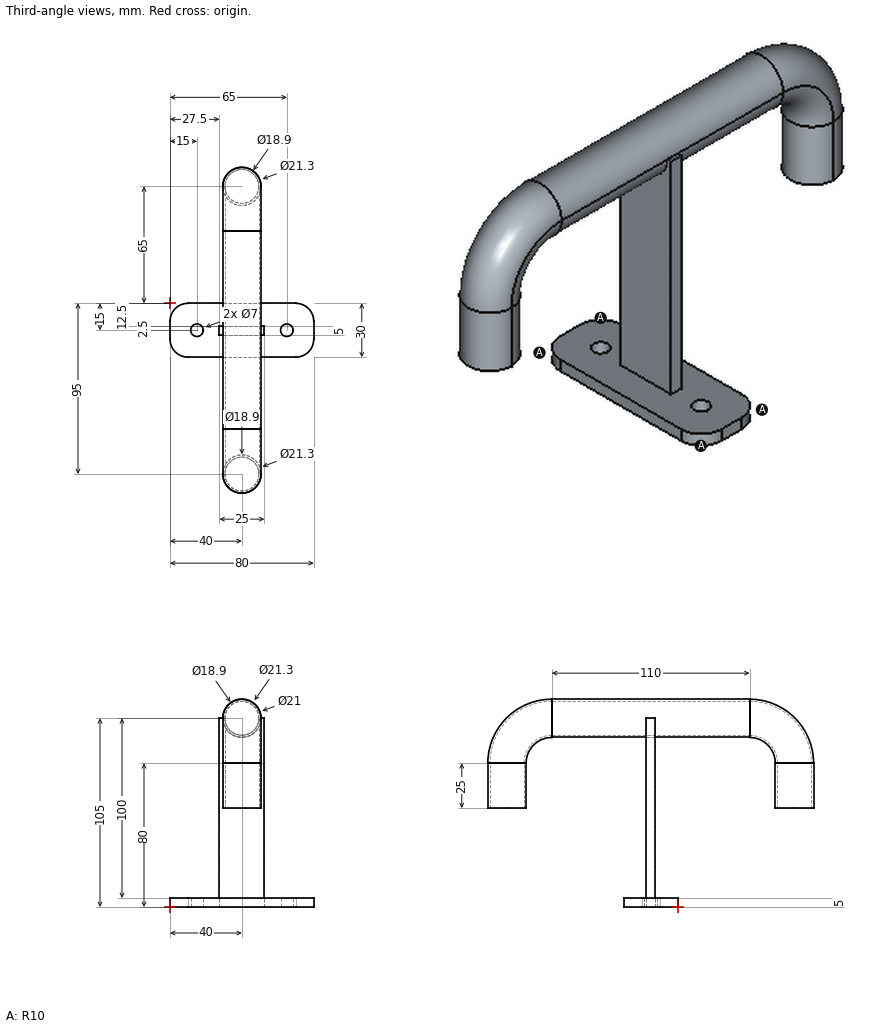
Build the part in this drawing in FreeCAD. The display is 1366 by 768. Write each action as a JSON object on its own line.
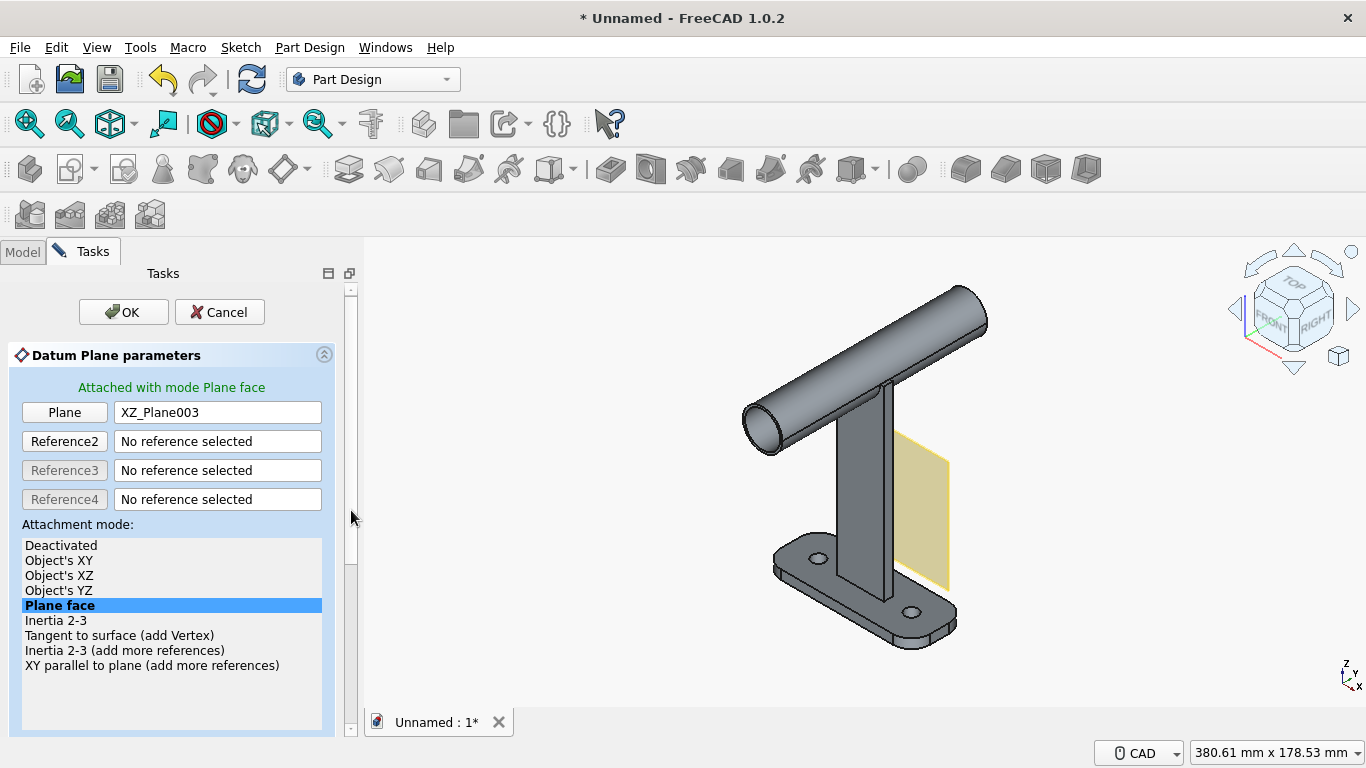
{"action": "left_click", "coordinate": [124, 312]}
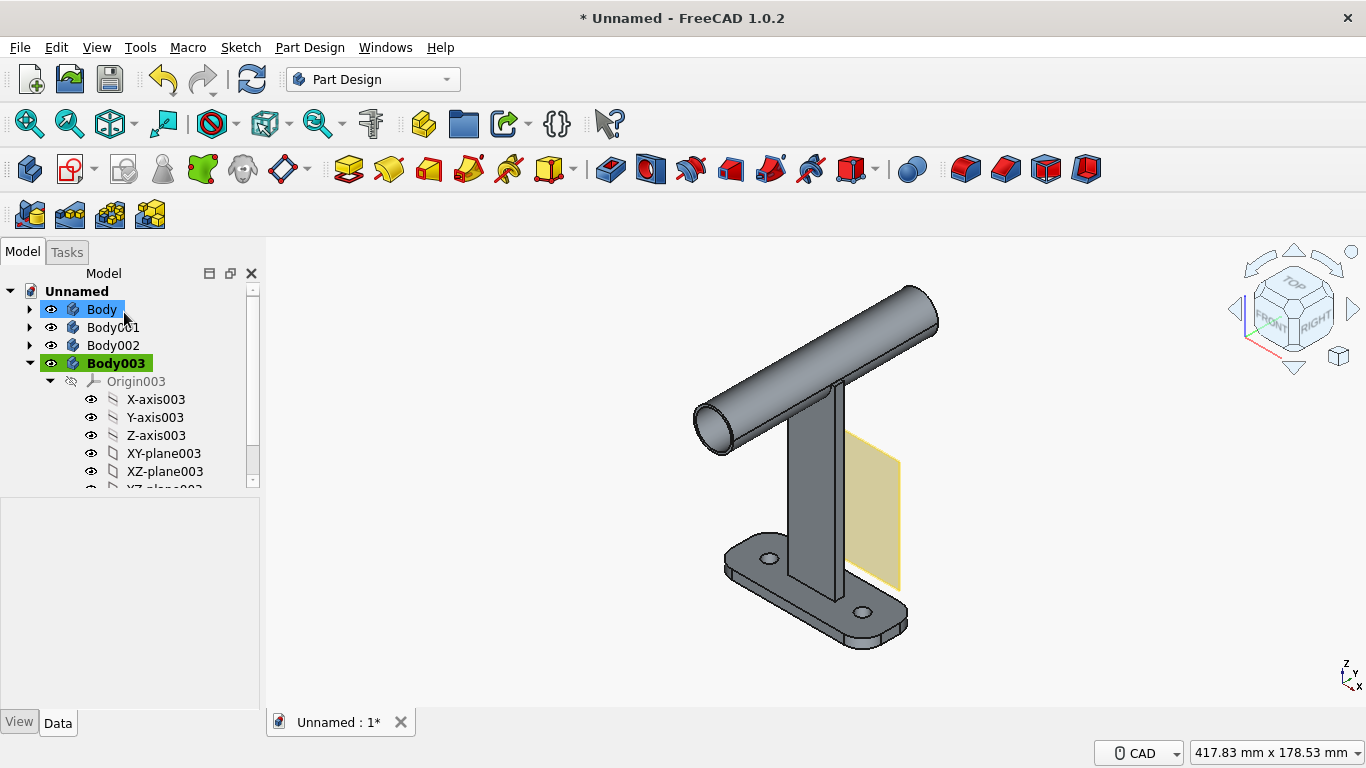
{"action": "scroll", "coordinate": [100, 377], "scroll_direction": "down", "scroll_amount": 3}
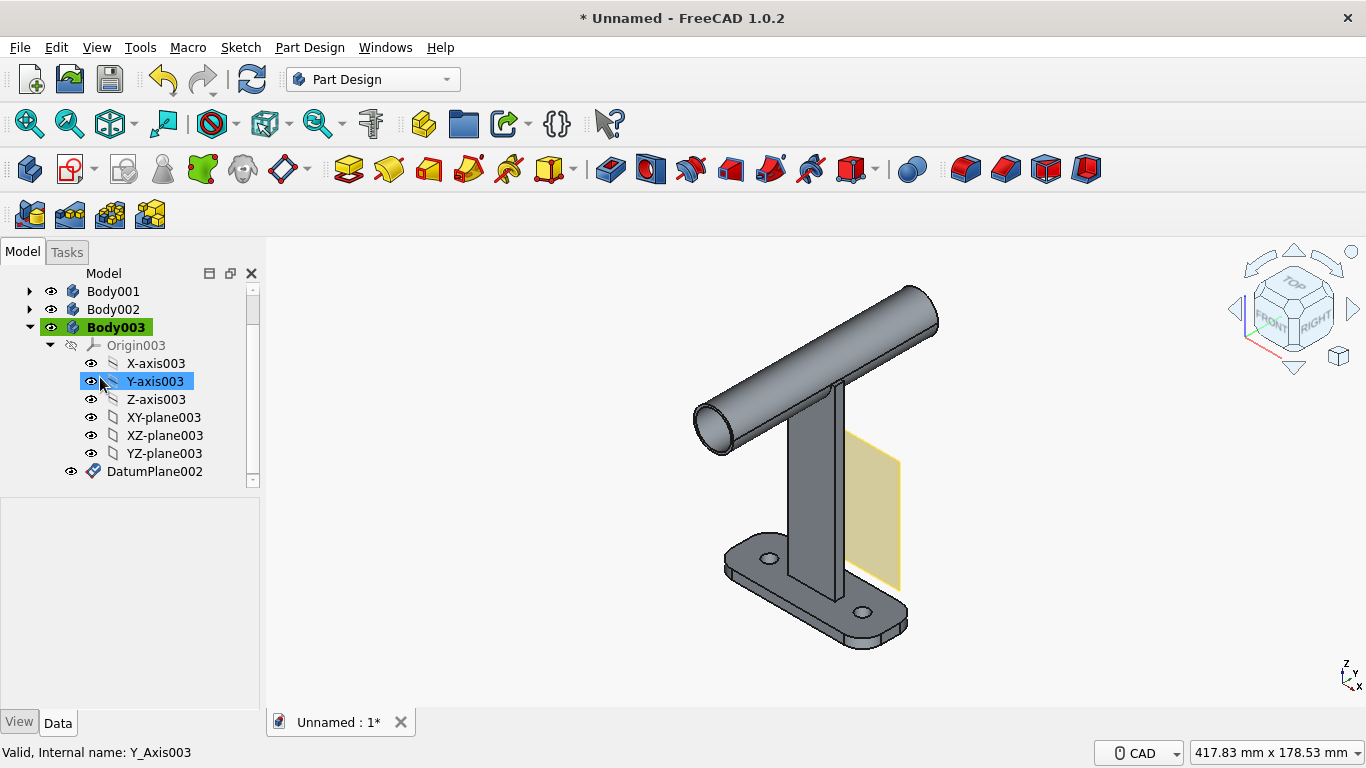
{"action": "left_click", "coordinate": [116, 471]}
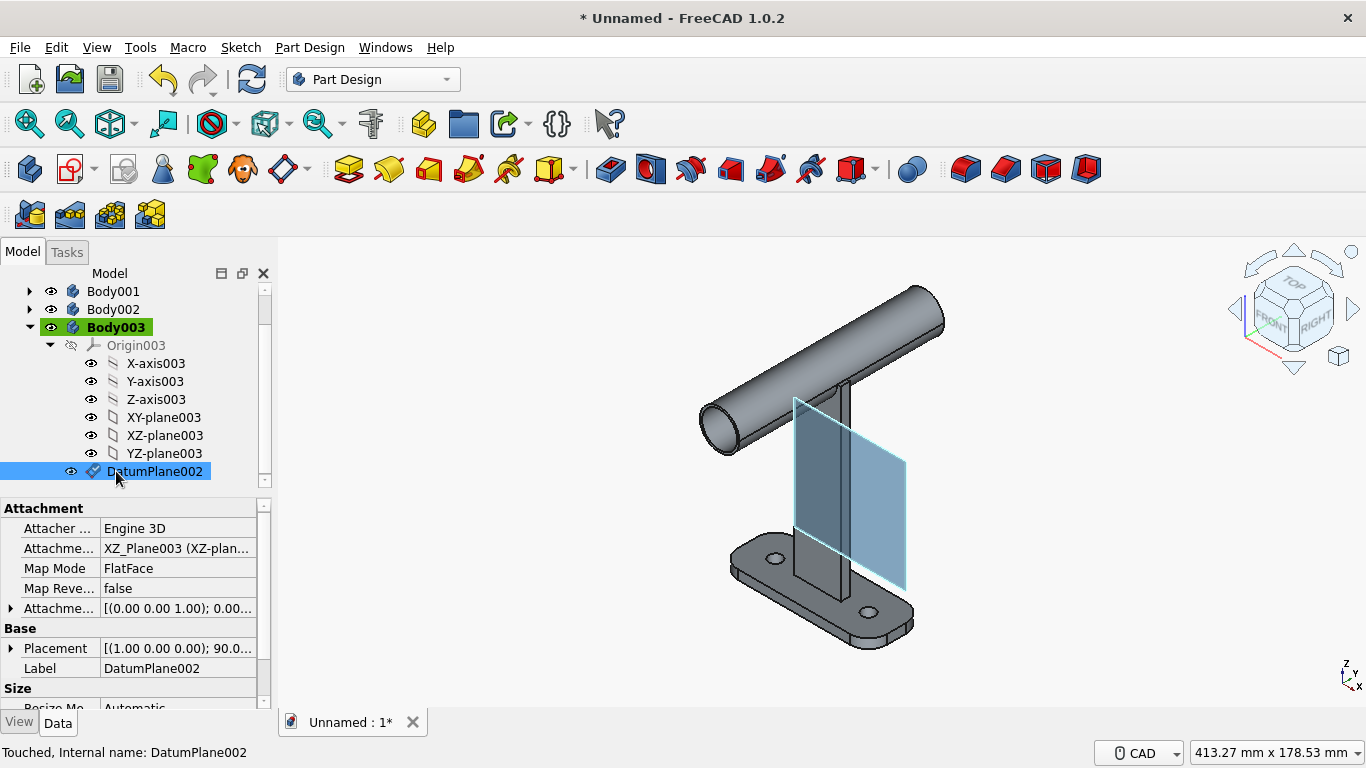
{"action": "left_click", "coordinate": [70, 170]}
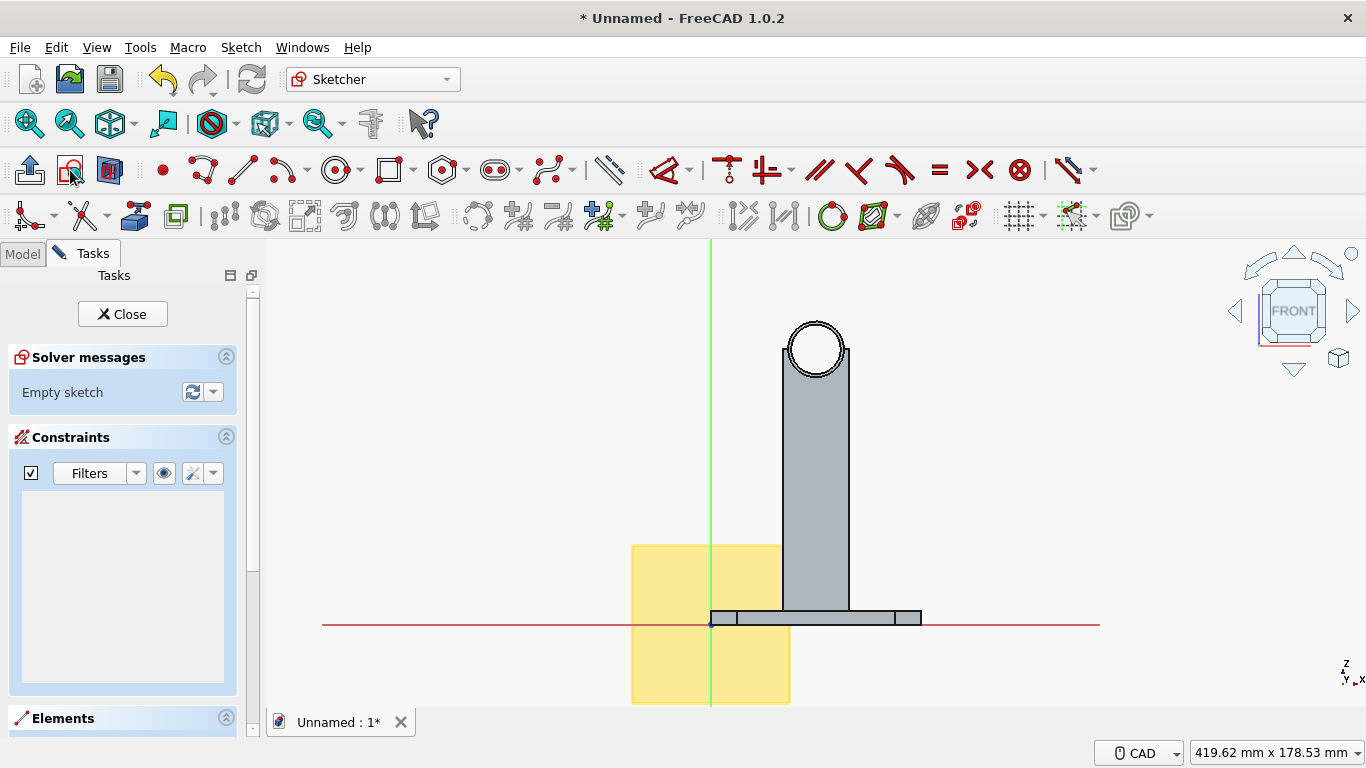
{"action": "scroll", "coordinate": [846, 323], "scroll_direction": "up", "scroll_amount": 6}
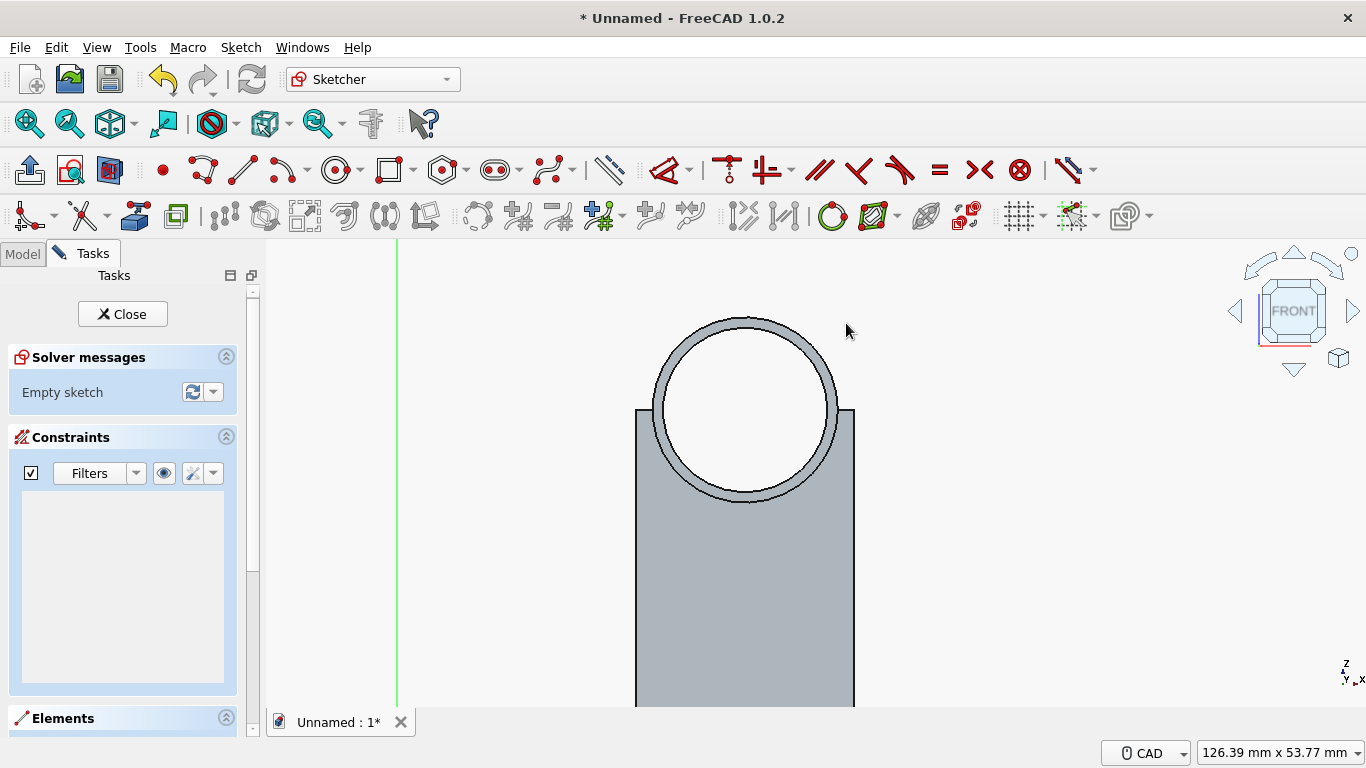
{"action": "left_click", "coordinate": [336, 170]}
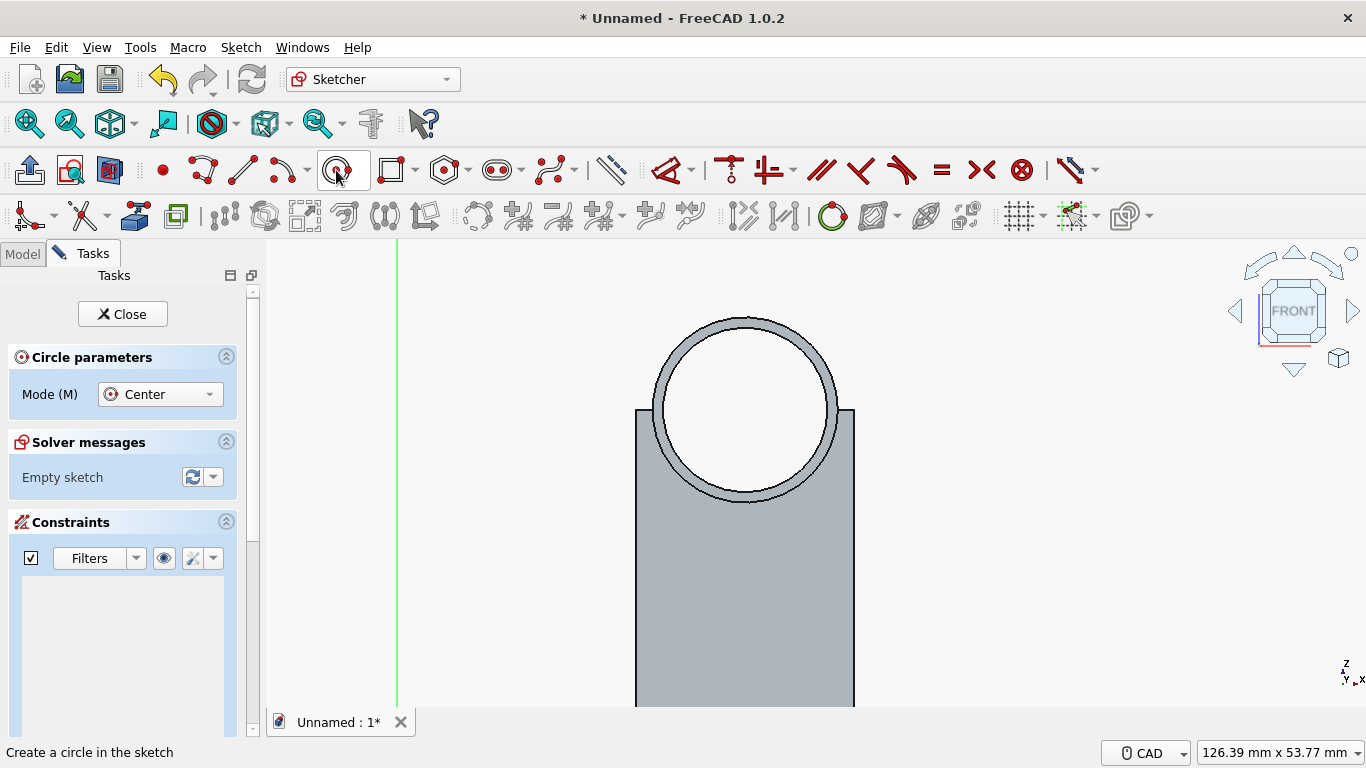
{"action": "left_click", "coordinate": [745, 410]}
{"action": "mouse_move", "coordinate": [811, 344]}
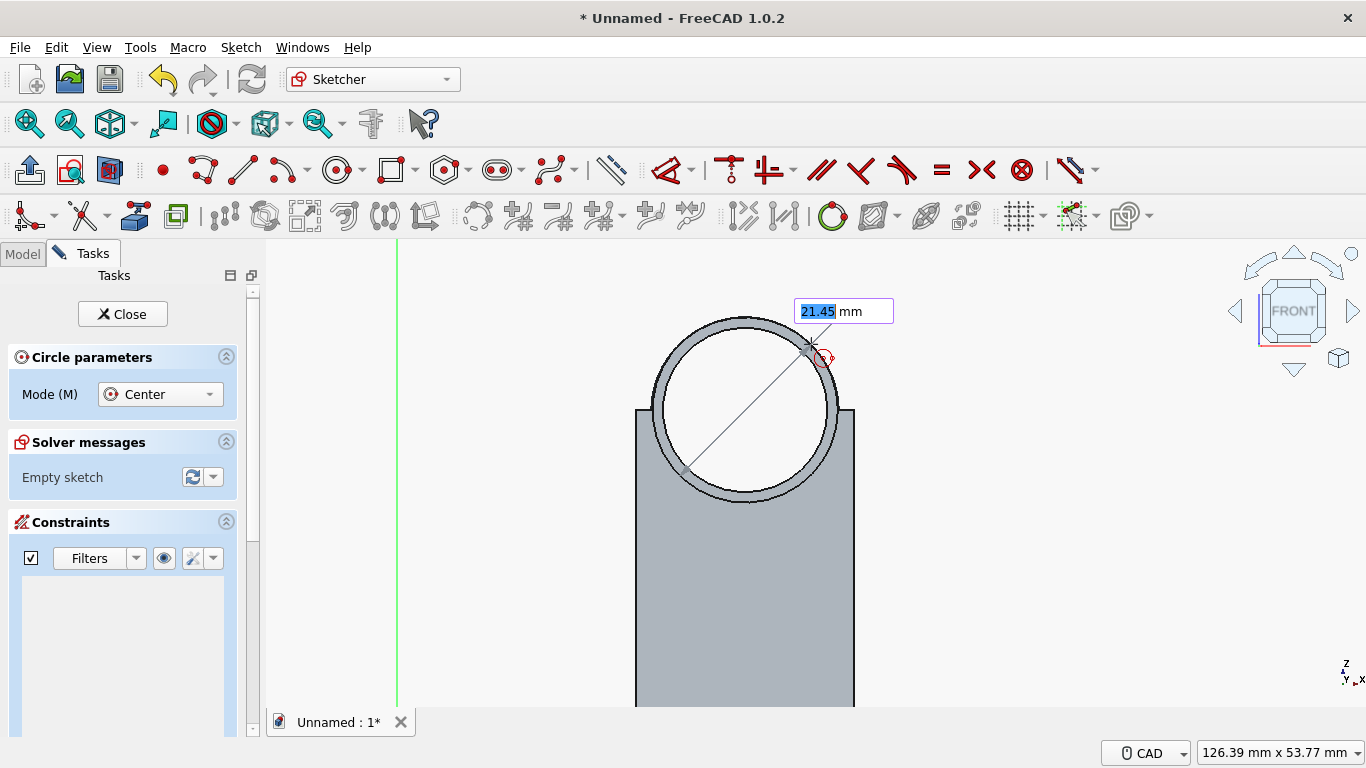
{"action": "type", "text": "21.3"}
{"action": "key", "text": "Return"}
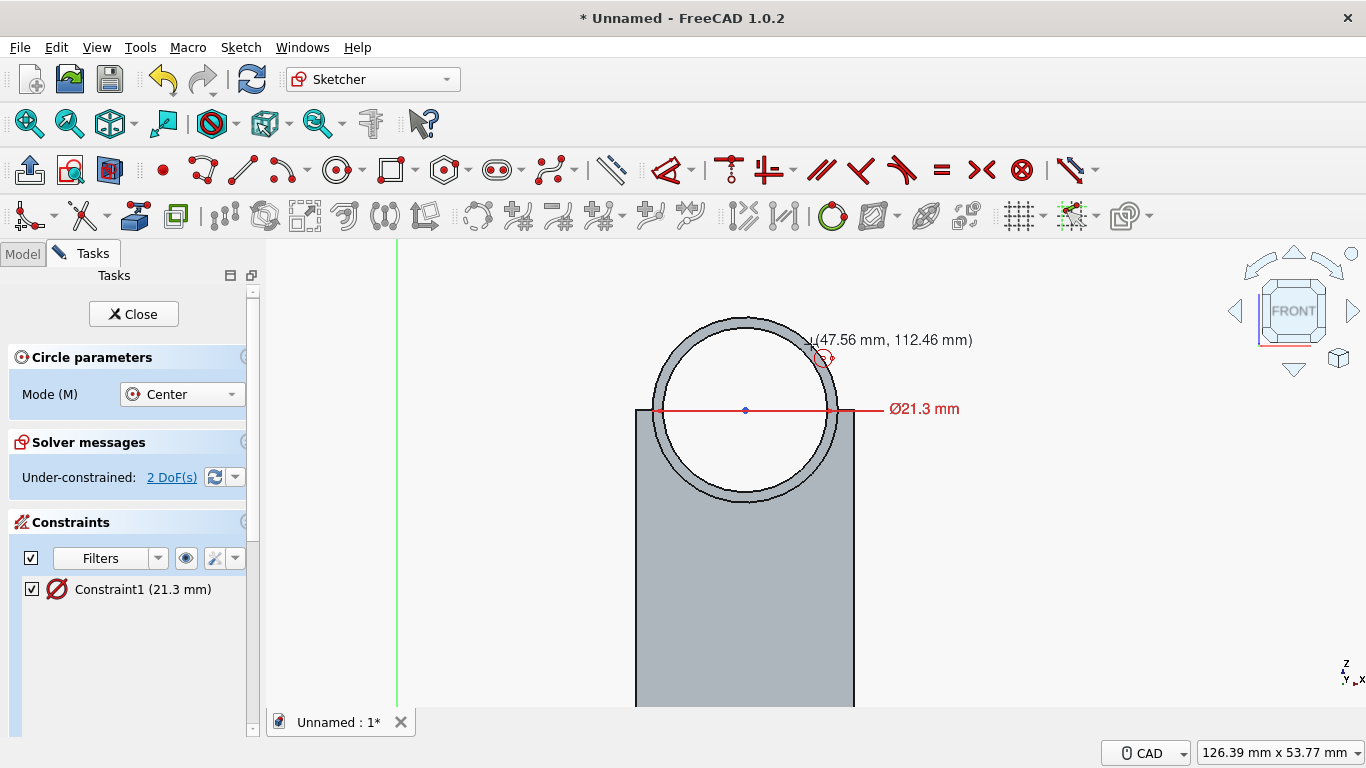
{"action": "left_click", "coordinate": [745, 411]}